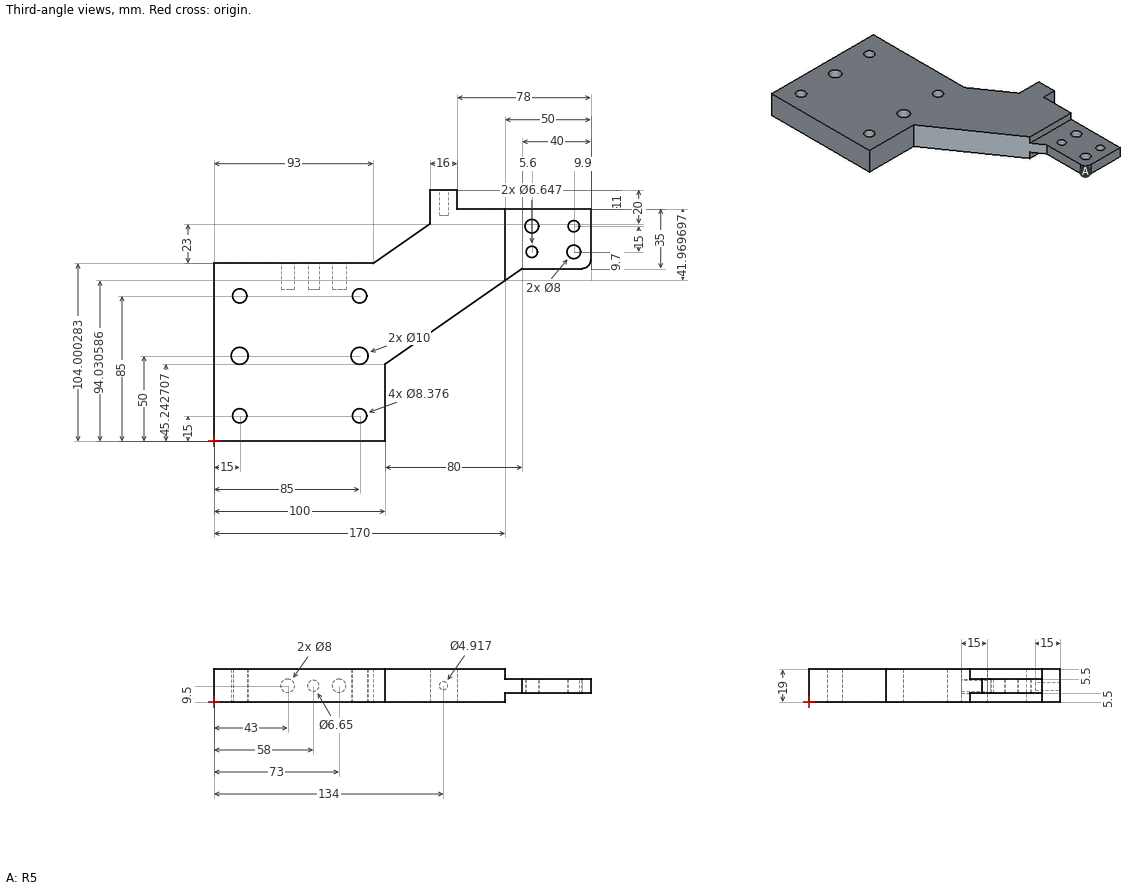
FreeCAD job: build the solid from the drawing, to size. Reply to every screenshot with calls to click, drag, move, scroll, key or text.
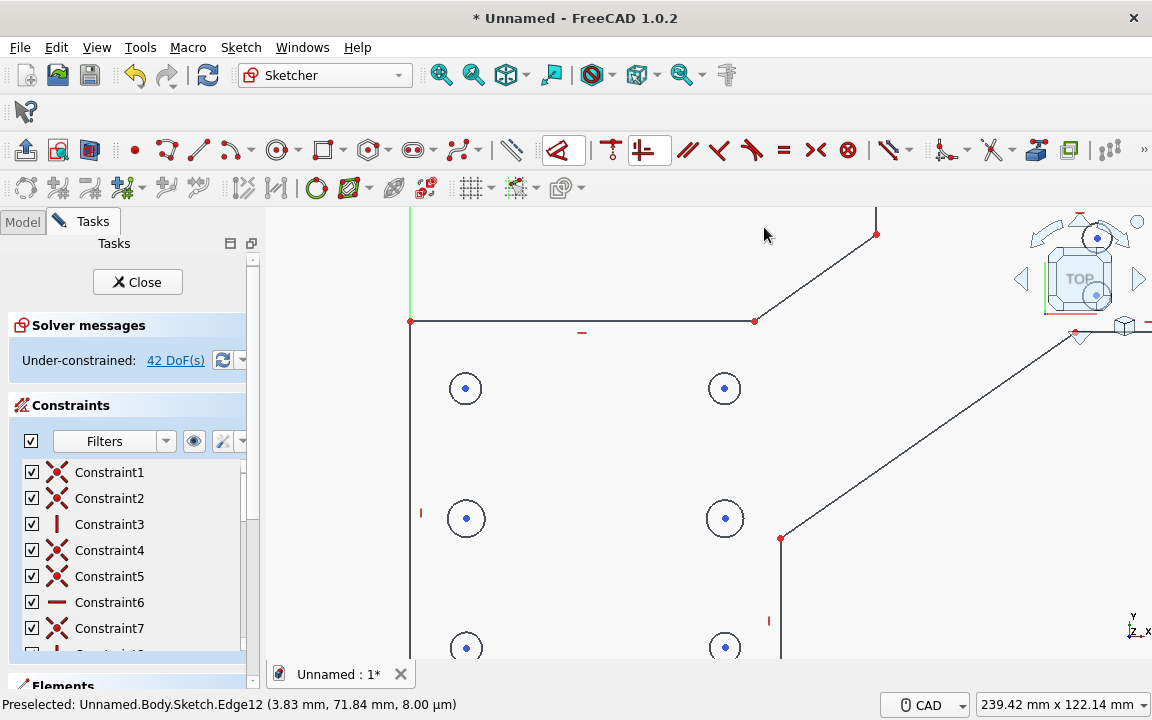
scroll(425, 436, down, 3)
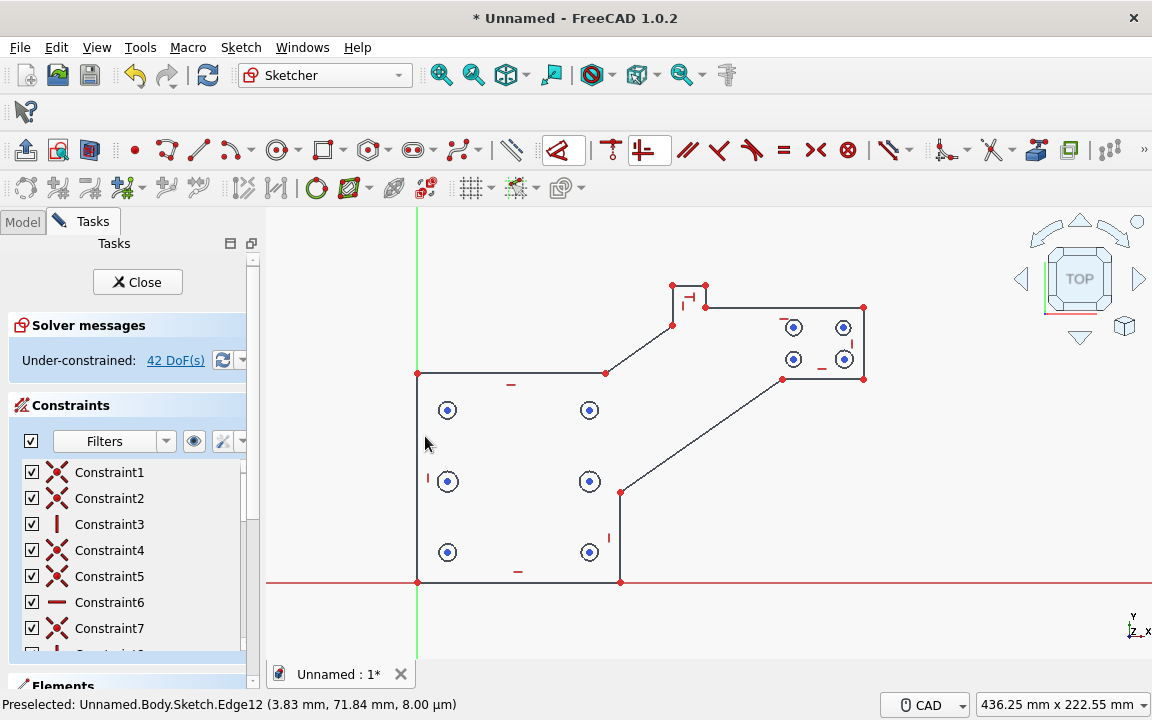
scroll(596, 547, up, 3)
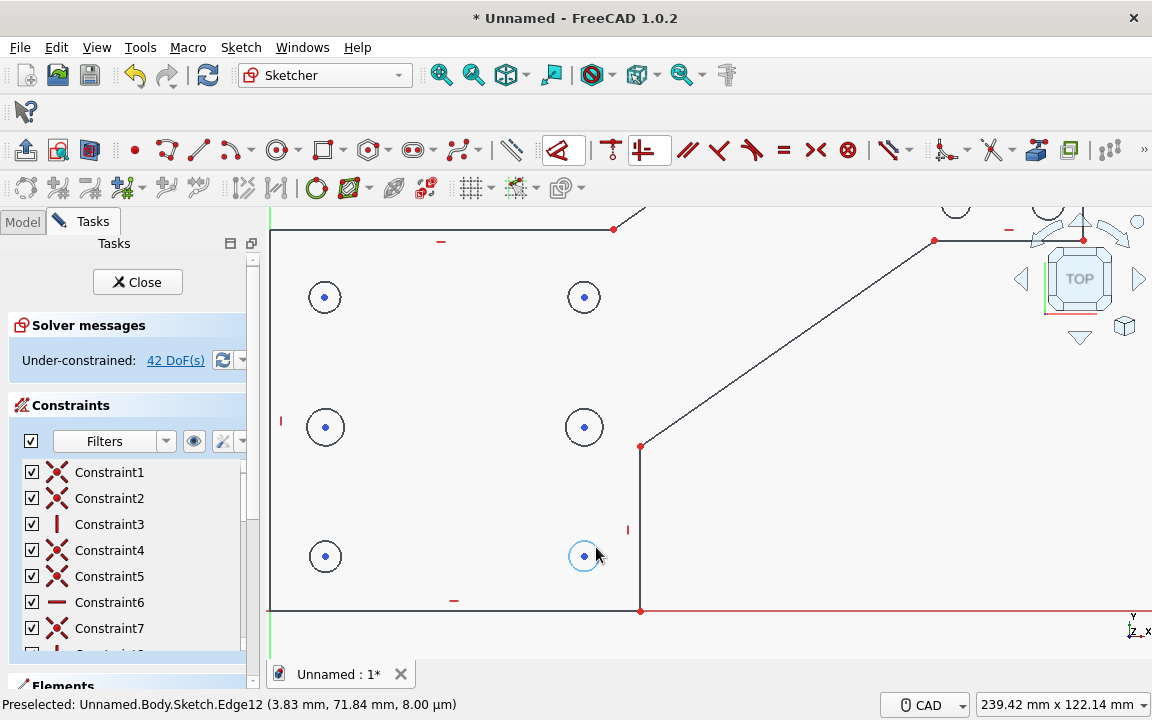
click(595, 545)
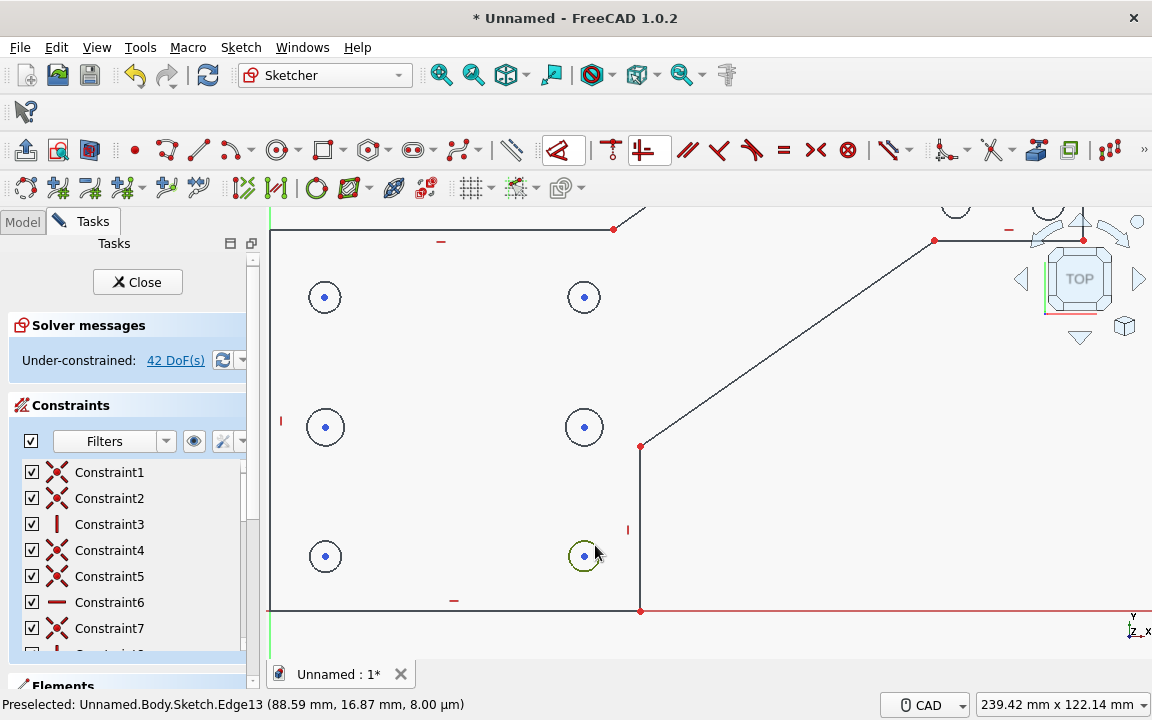
click(337, 546)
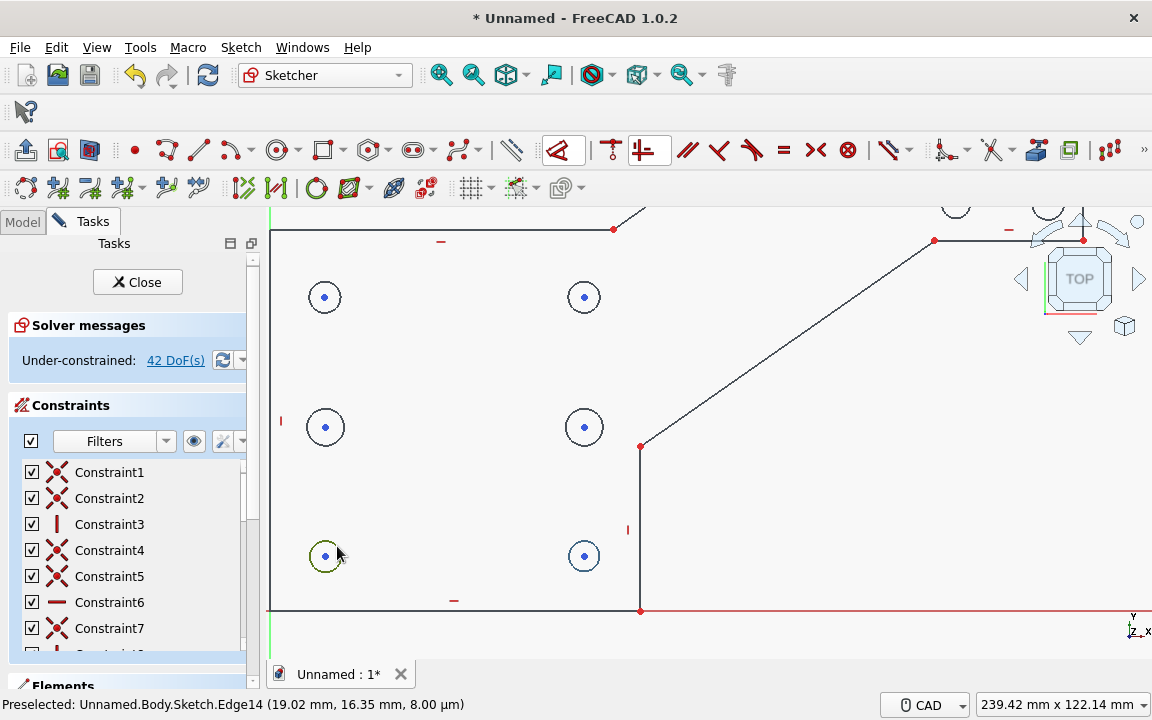
click(595, 286)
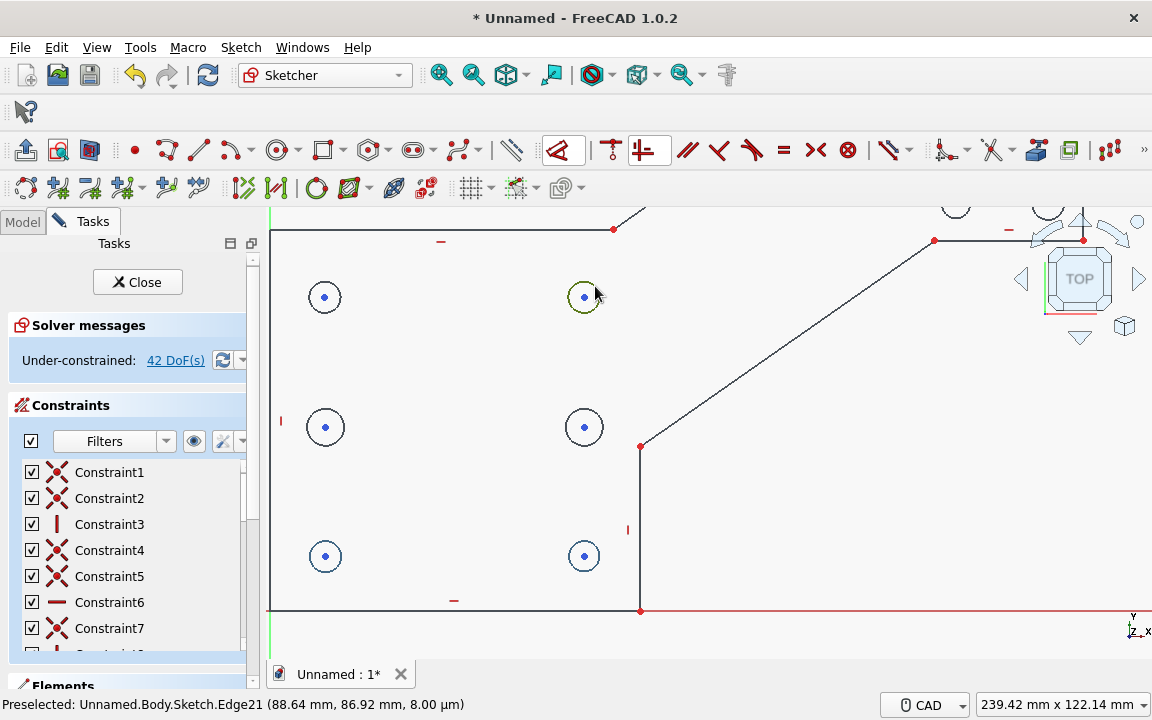
click(336, 286)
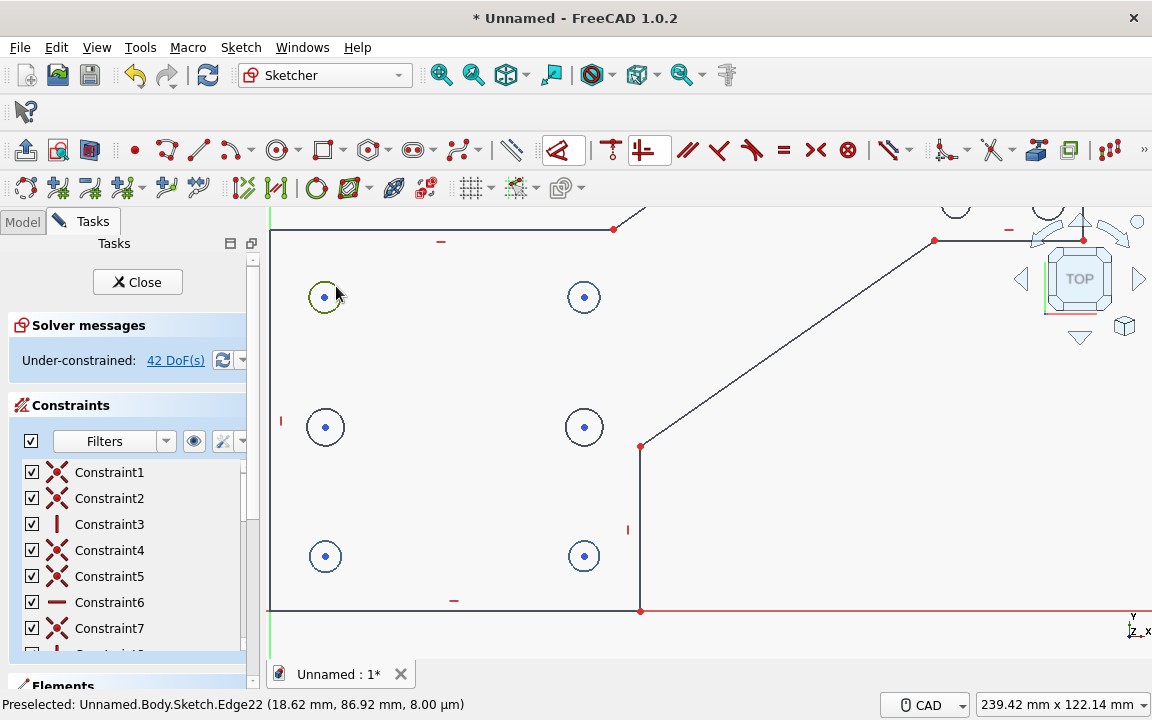
click(784, 150)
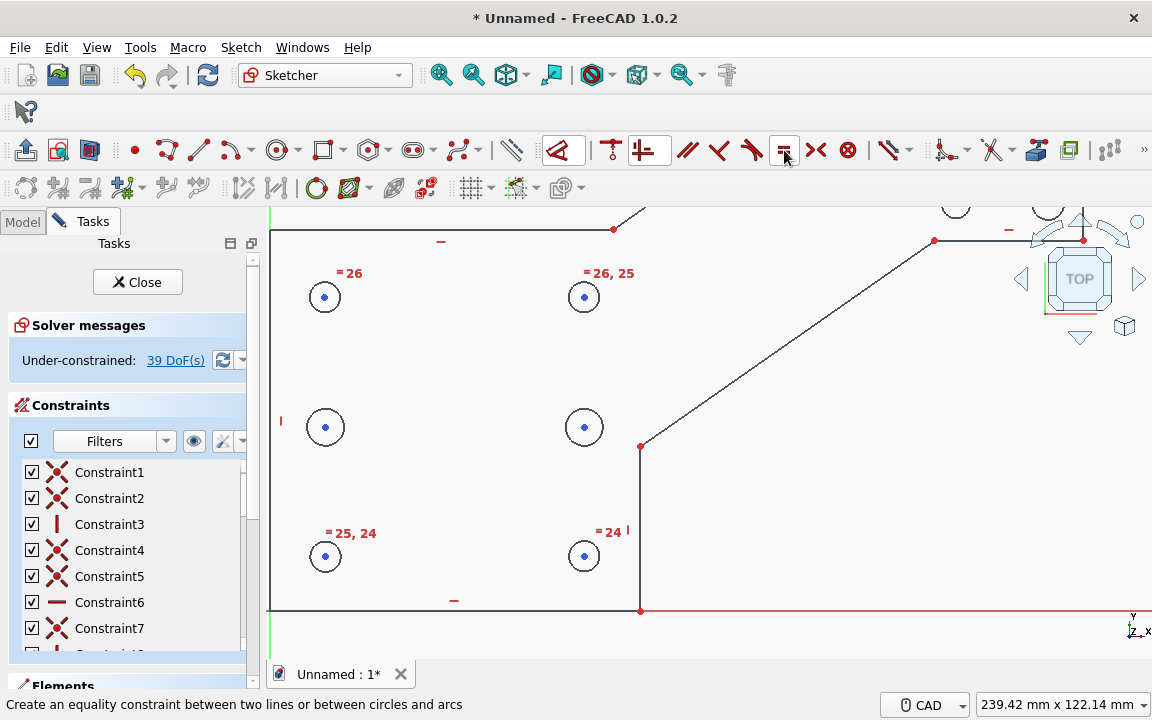
click(597, 414)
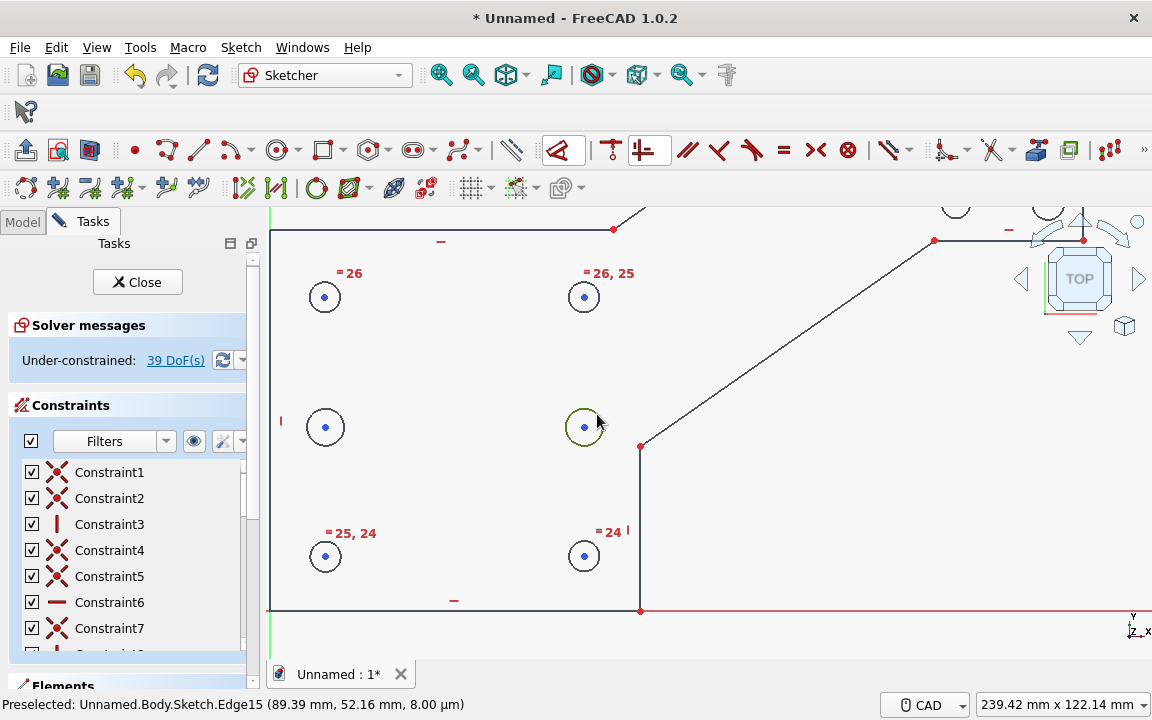
click(339, 414)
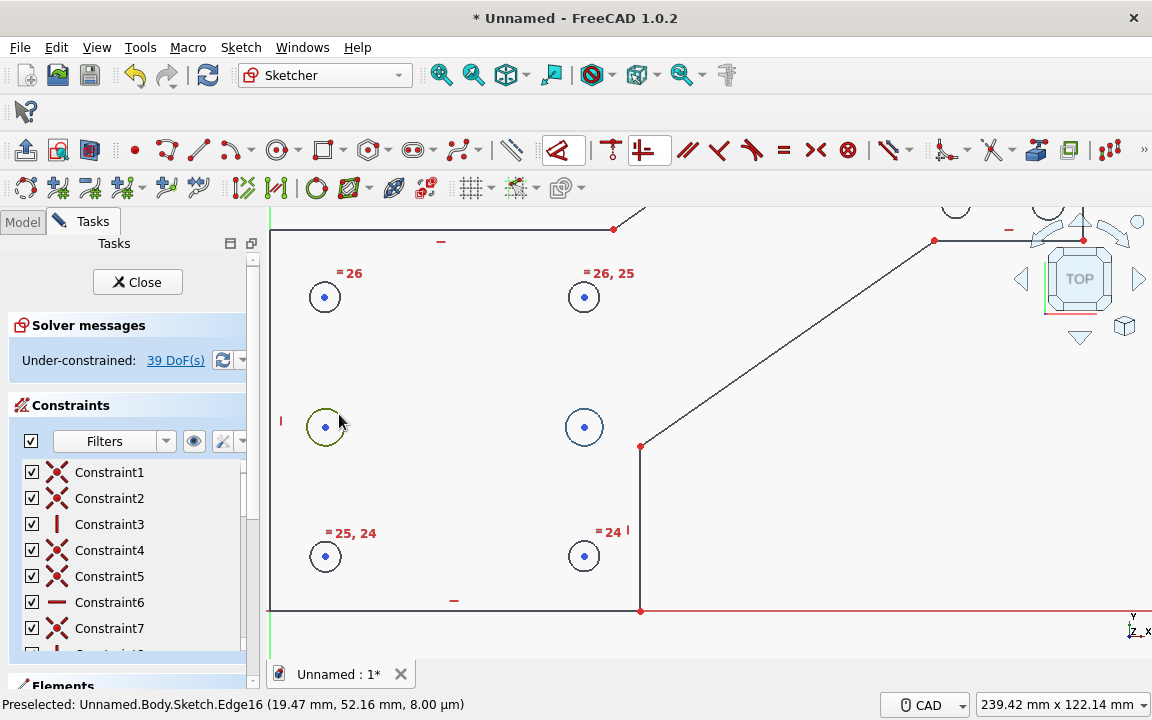
click(784, 150)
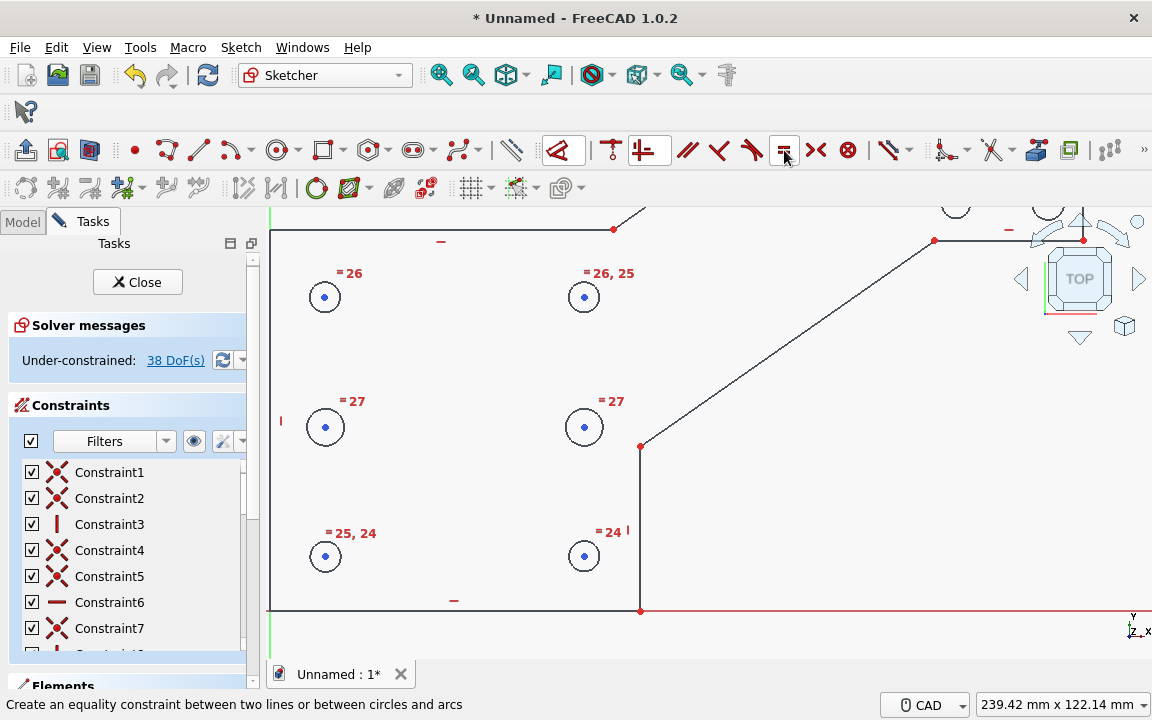
scroll(596, 547, down, 3)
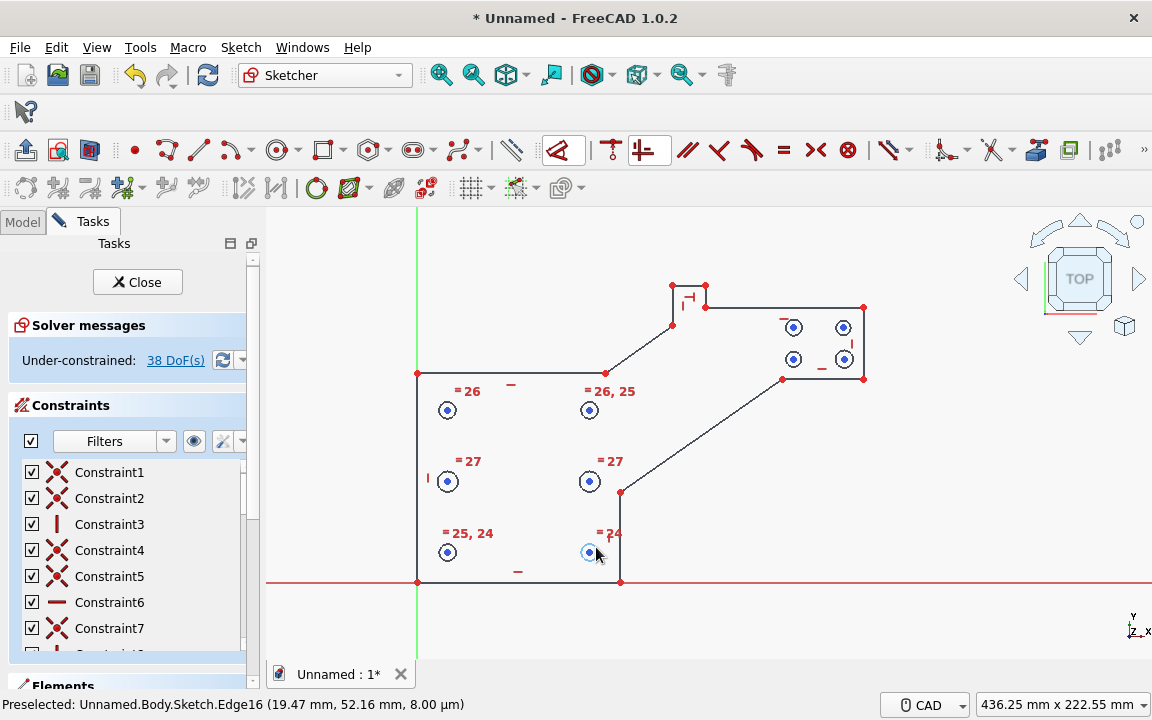
scroll(799, 354, up, 3)